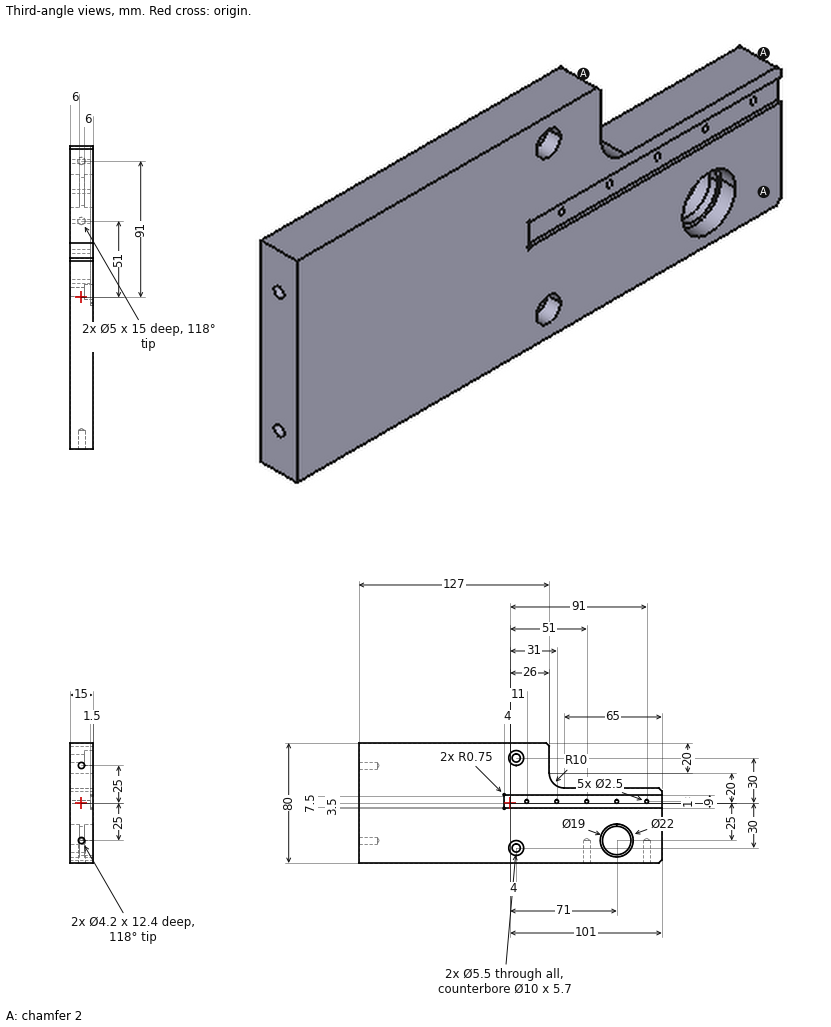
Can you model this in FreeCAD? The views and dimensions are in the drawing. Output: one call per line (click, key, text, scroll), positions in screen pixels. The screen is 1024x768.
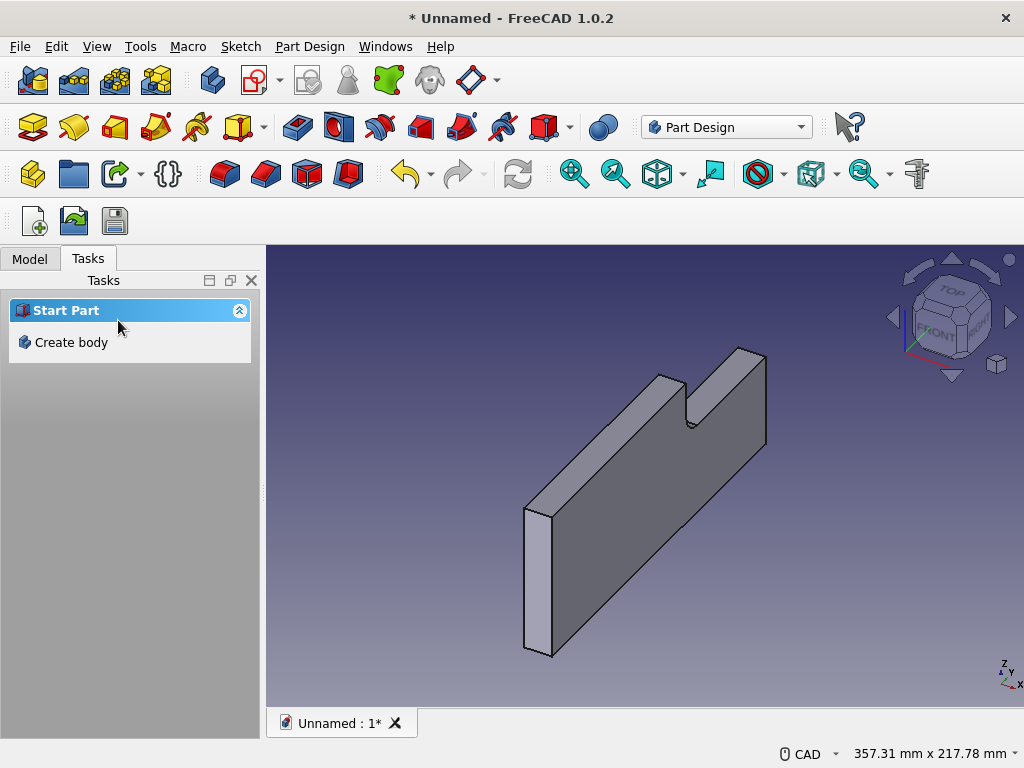
click(598, 540)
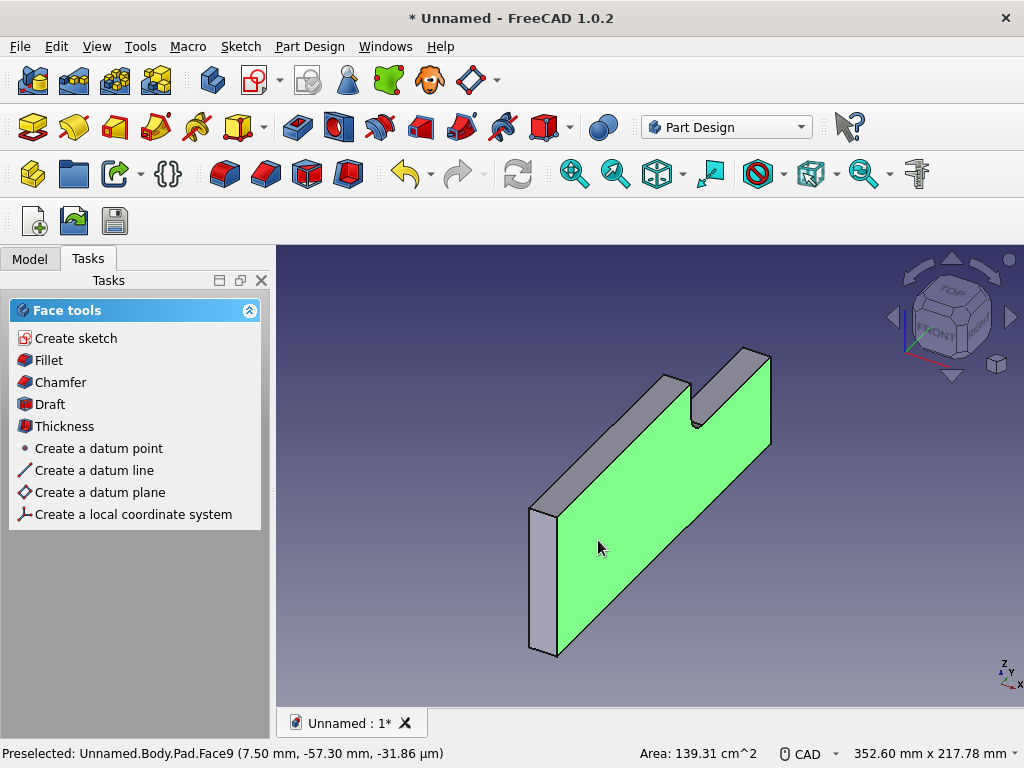
click(254, 80)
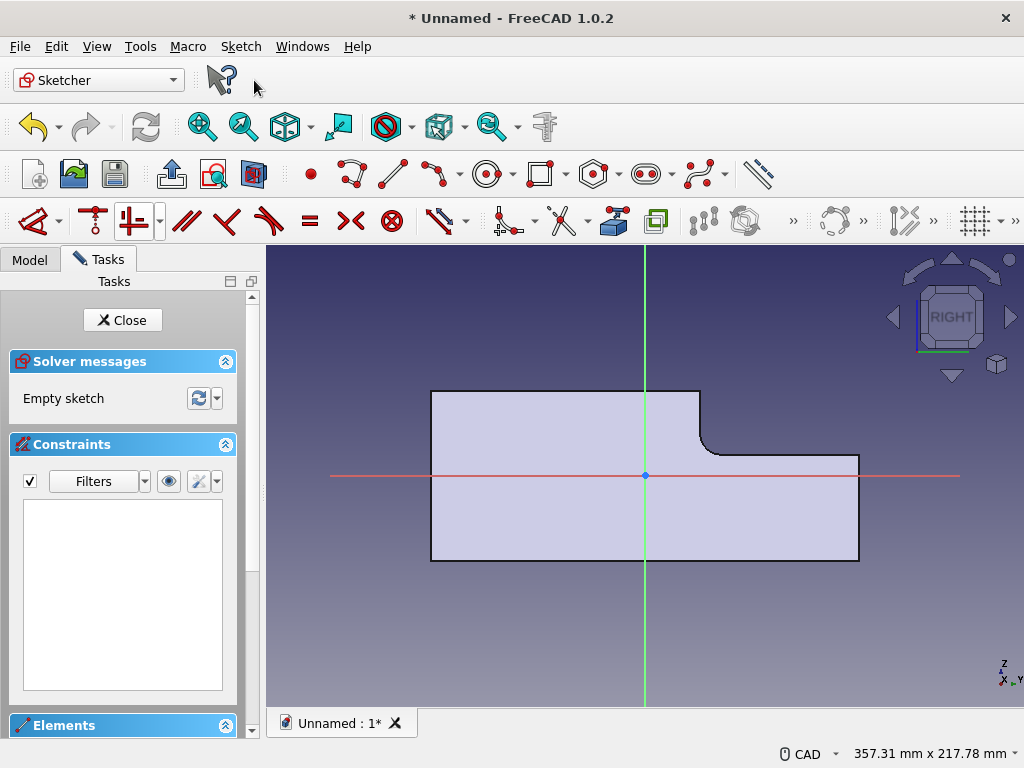
scroll(839, 540, up, 9)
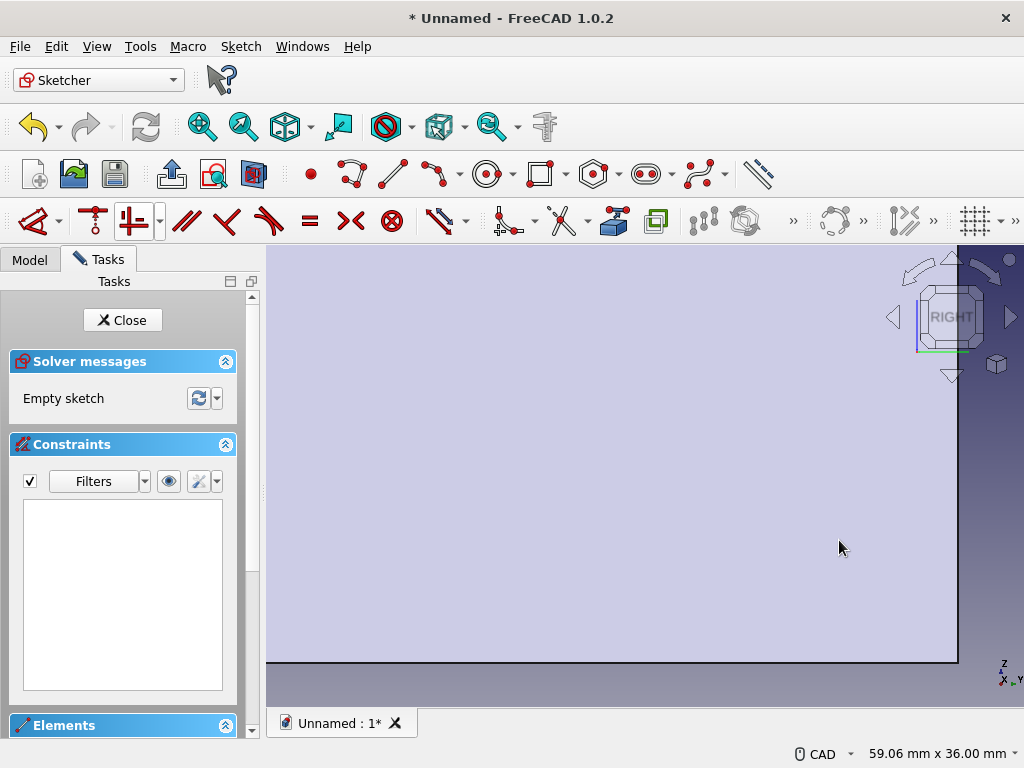
click(486, 174)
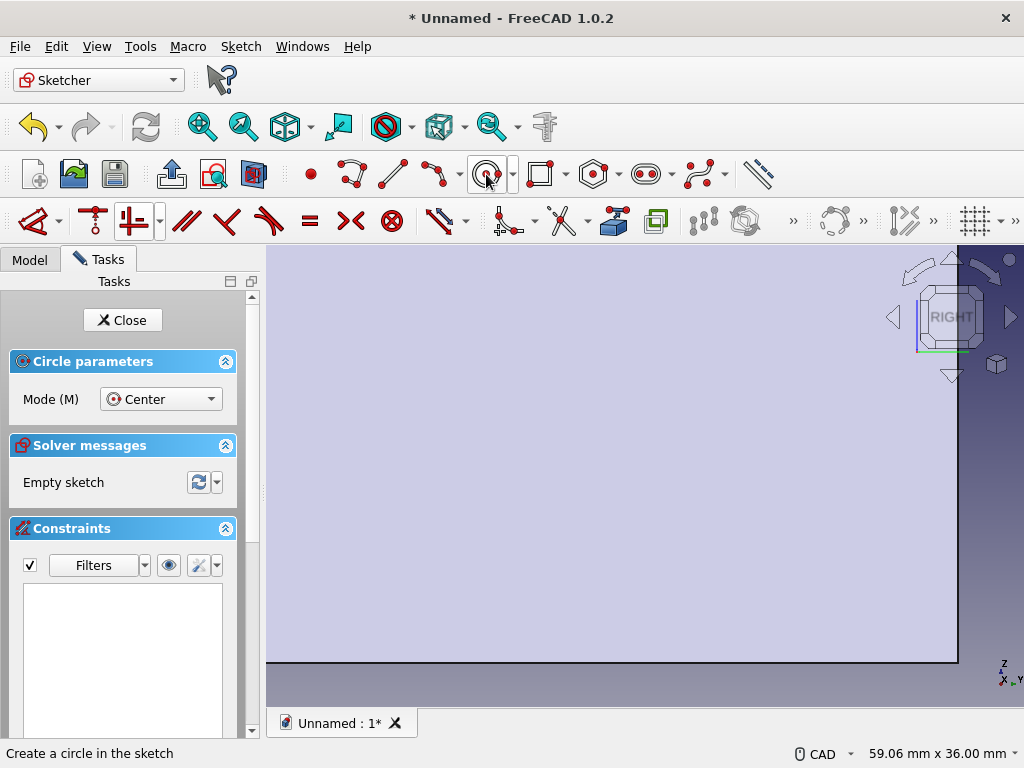
click(573, 470)
click(673, 371)
key(Escape)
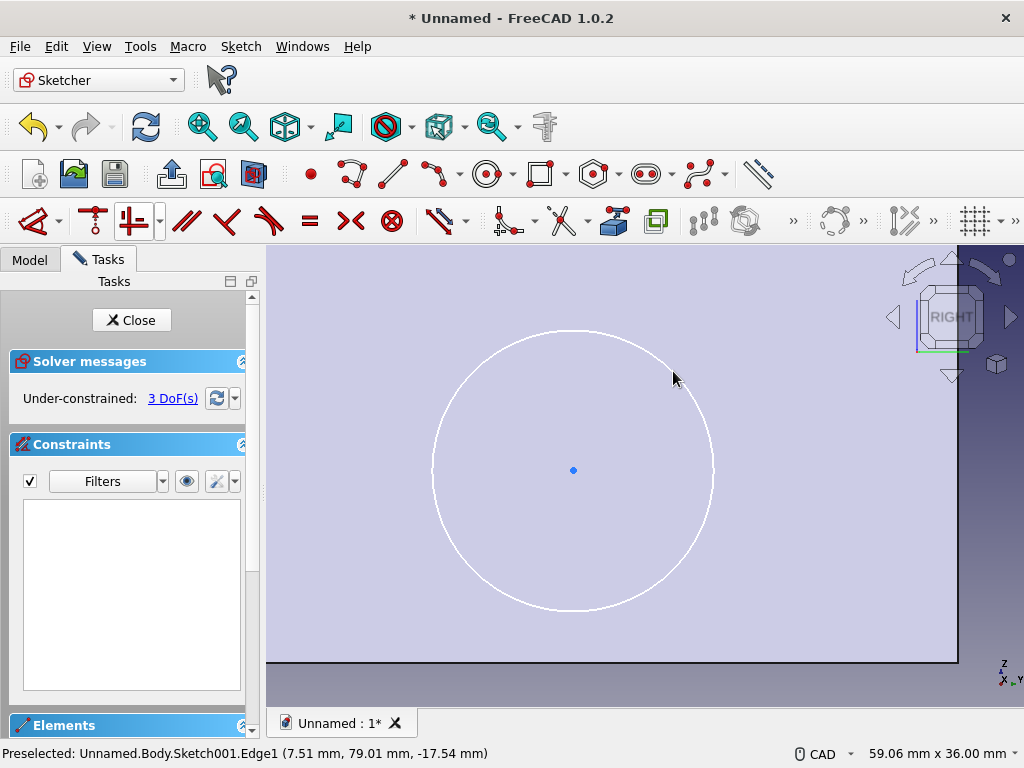
click(32, 222)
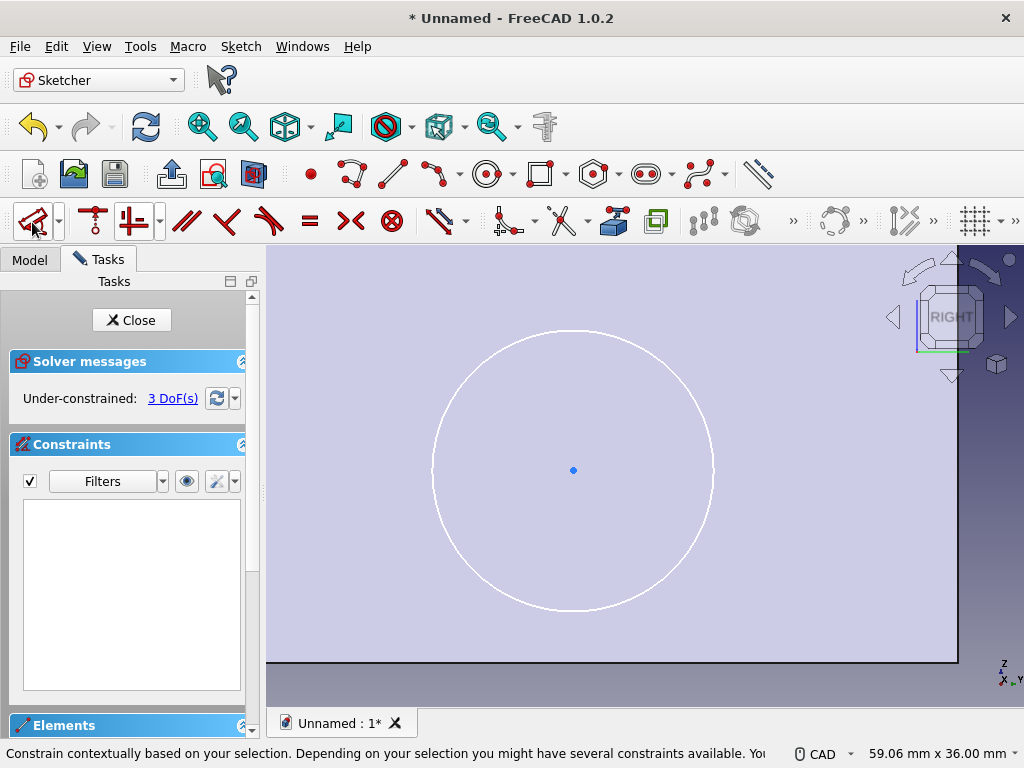
click(672, 371)
click(695, 348)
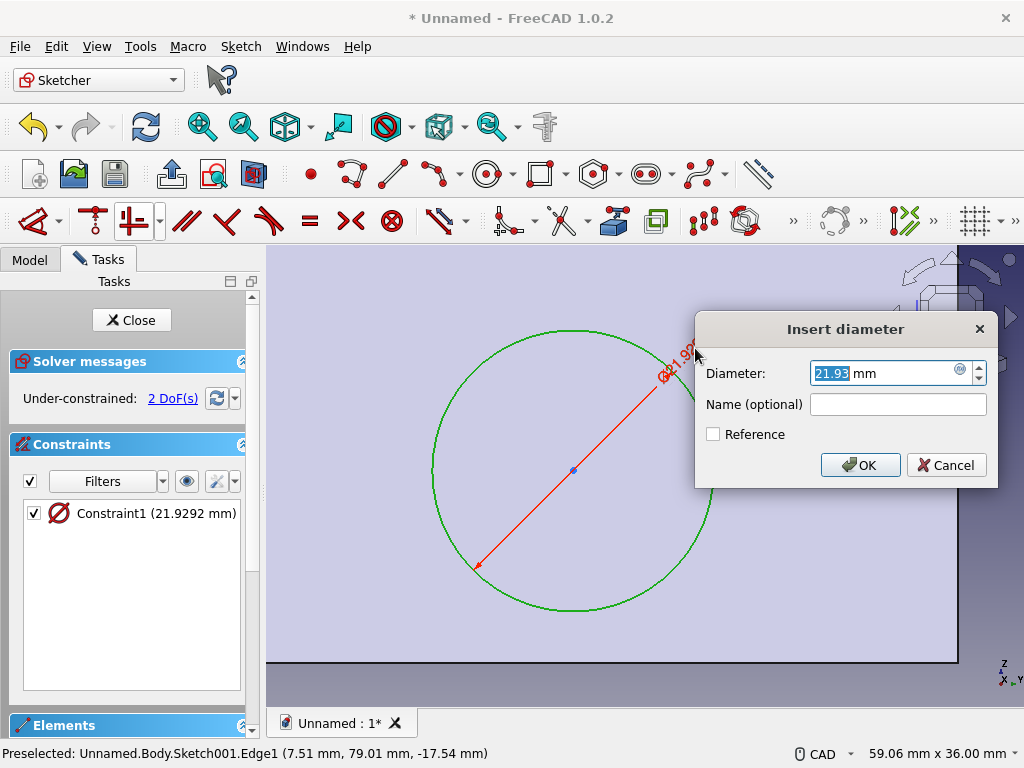
text(22)
key(Return)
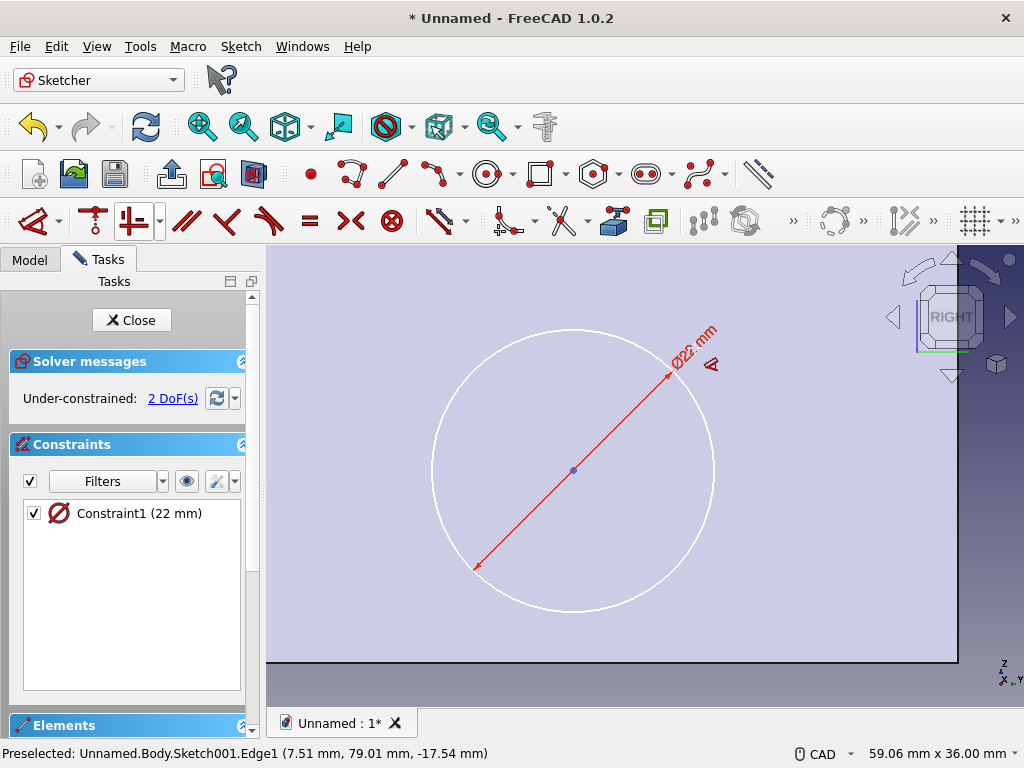
click(573, 471)
click(369, 505)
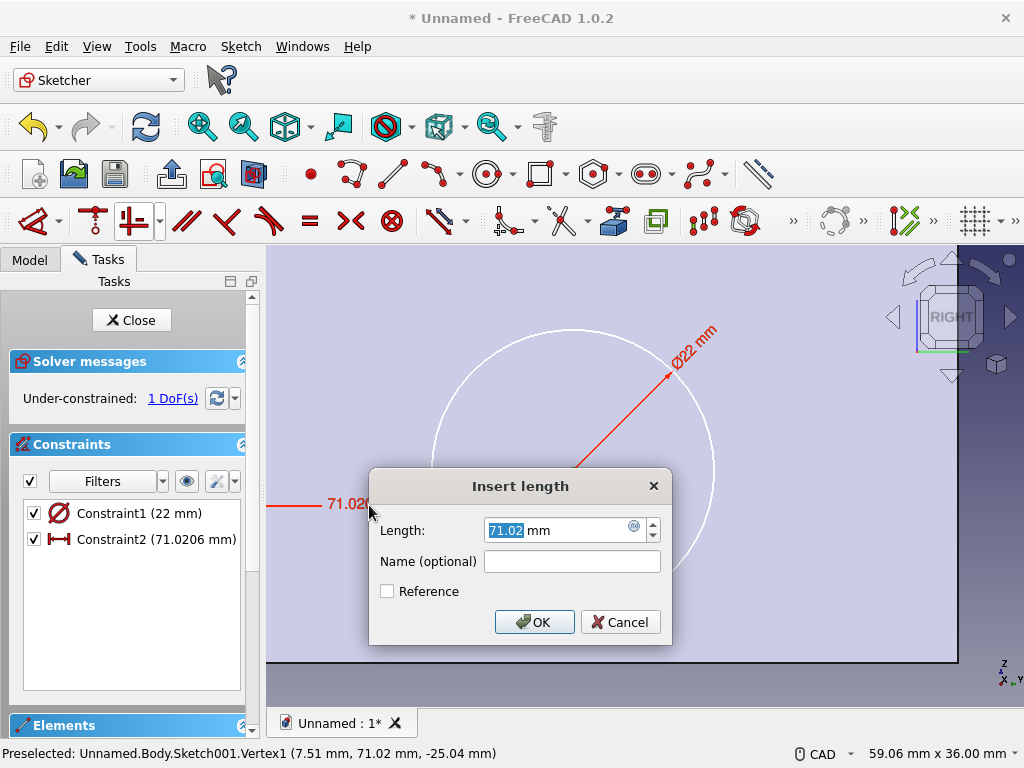
text(71)
key(Return)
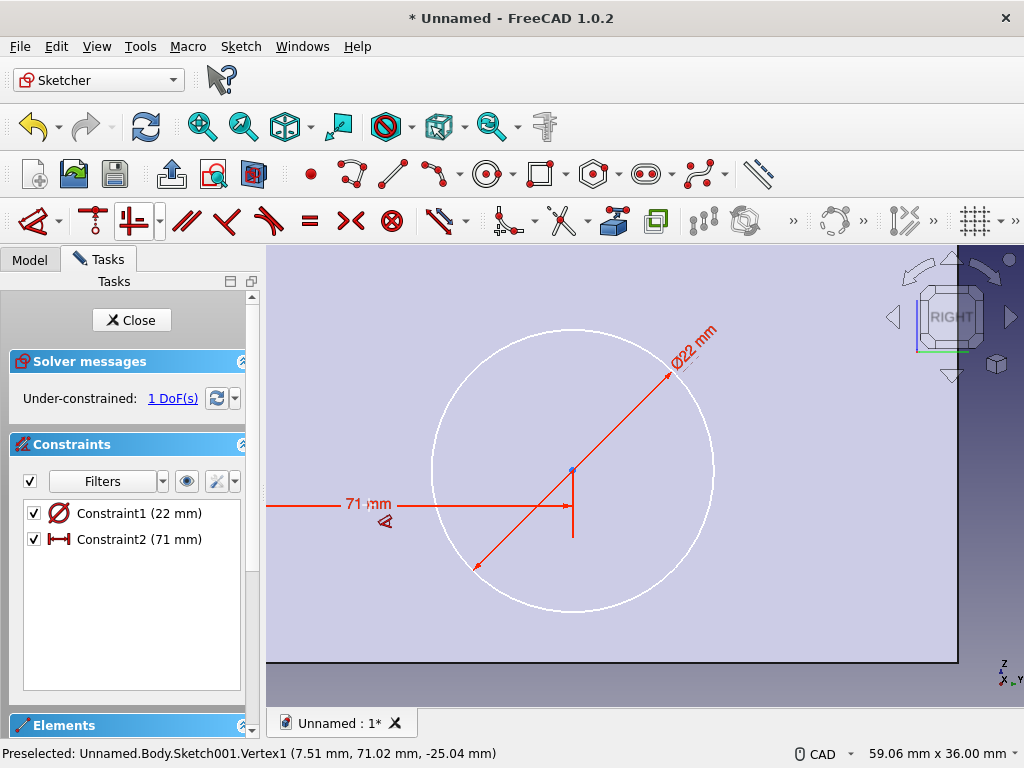
click(573, 471)
click(607, 372)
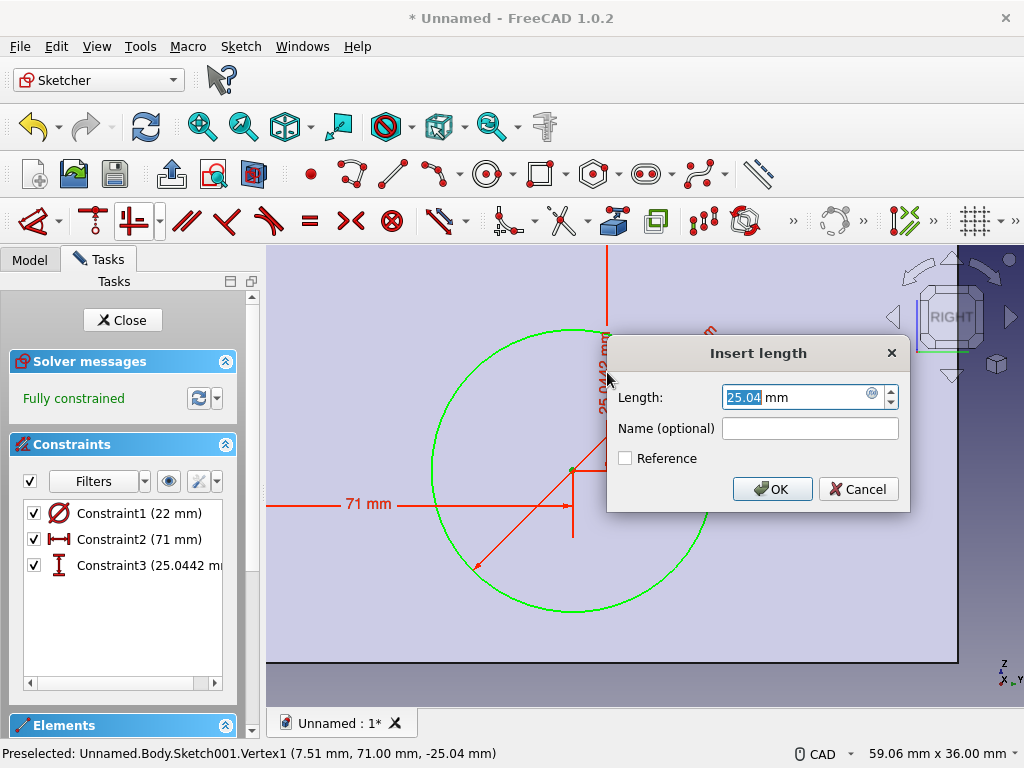
text(25)
key(Return)
key(Escape)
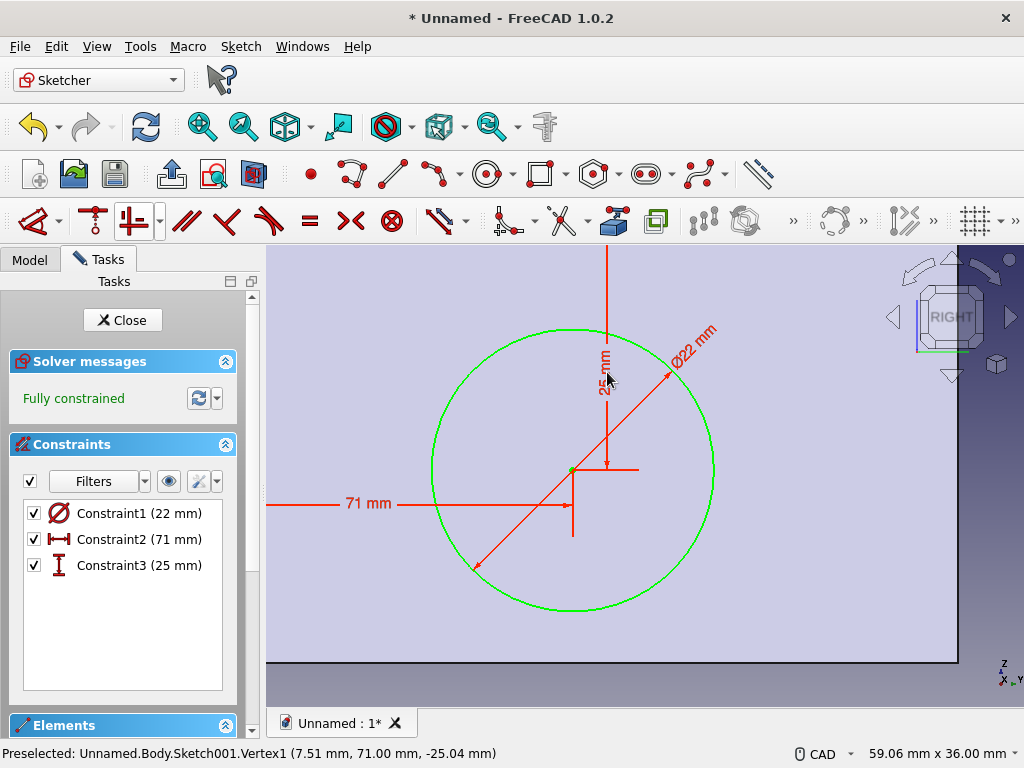
click(123, 320)